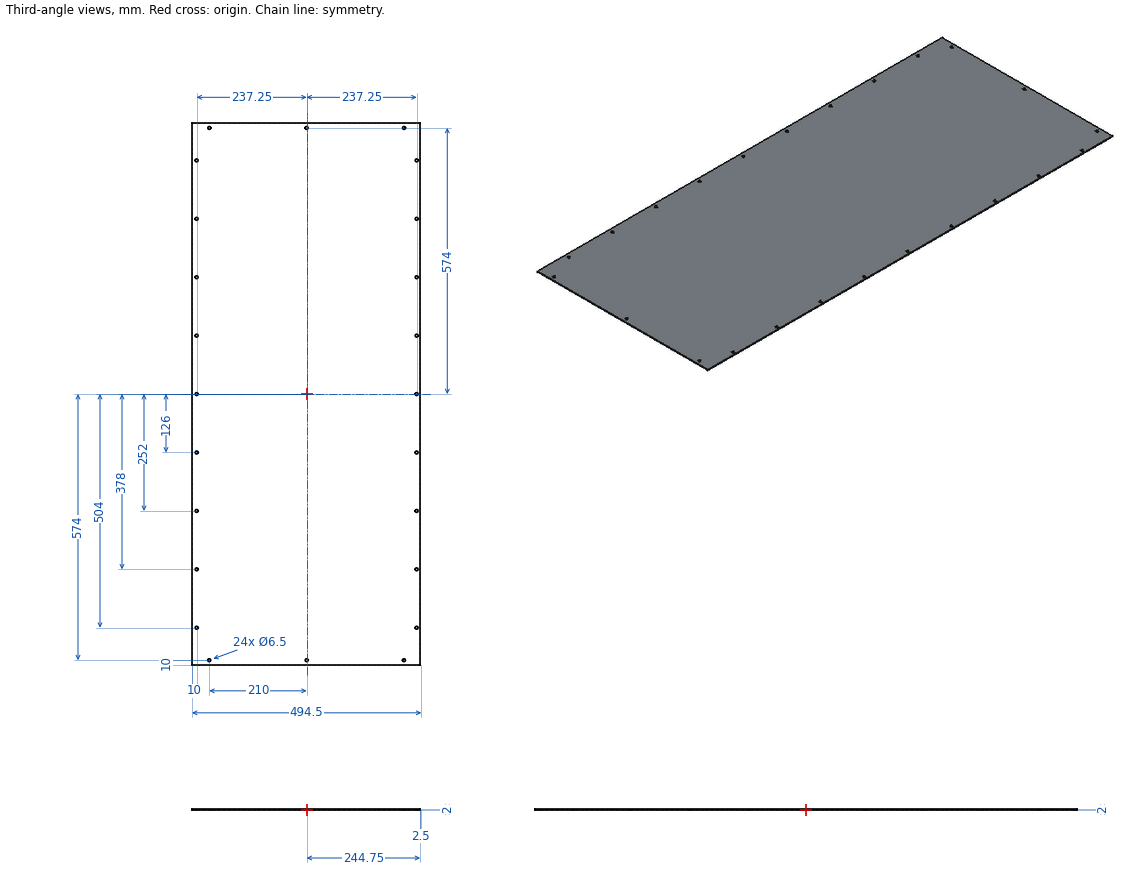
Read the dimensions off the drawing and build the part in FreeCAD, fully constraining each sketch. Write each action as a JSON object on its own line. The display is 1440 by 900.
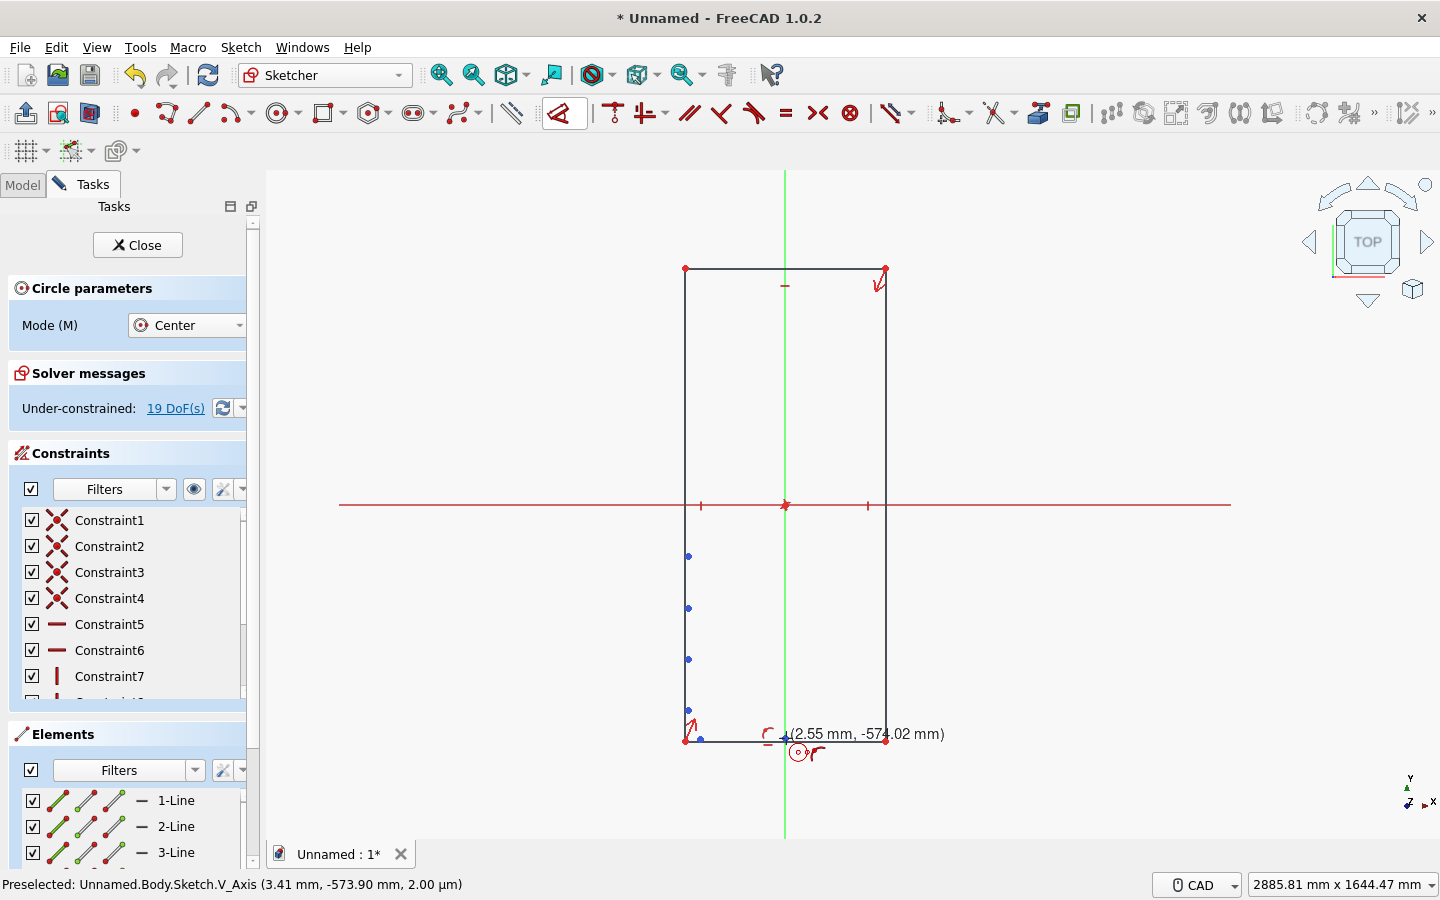
{"action": "scroll", "coordinate": [871, 739], "scroll_direction": "up", "scroll_amount": 15}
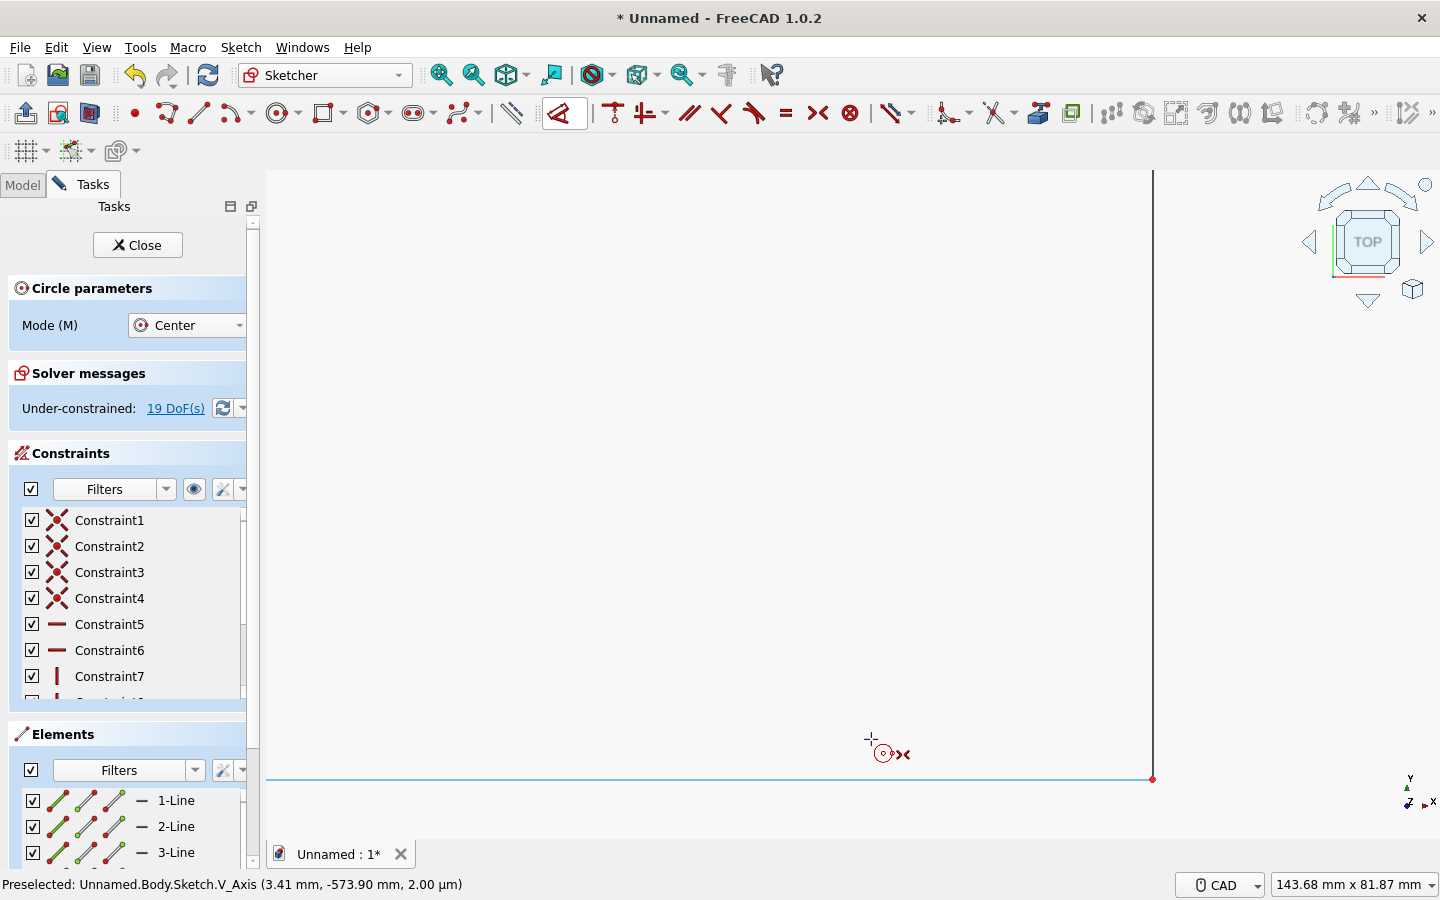
{"action": "scroll", "coordinate": [871, 739], "scroll_direction": "down", "scroll_amount": 15}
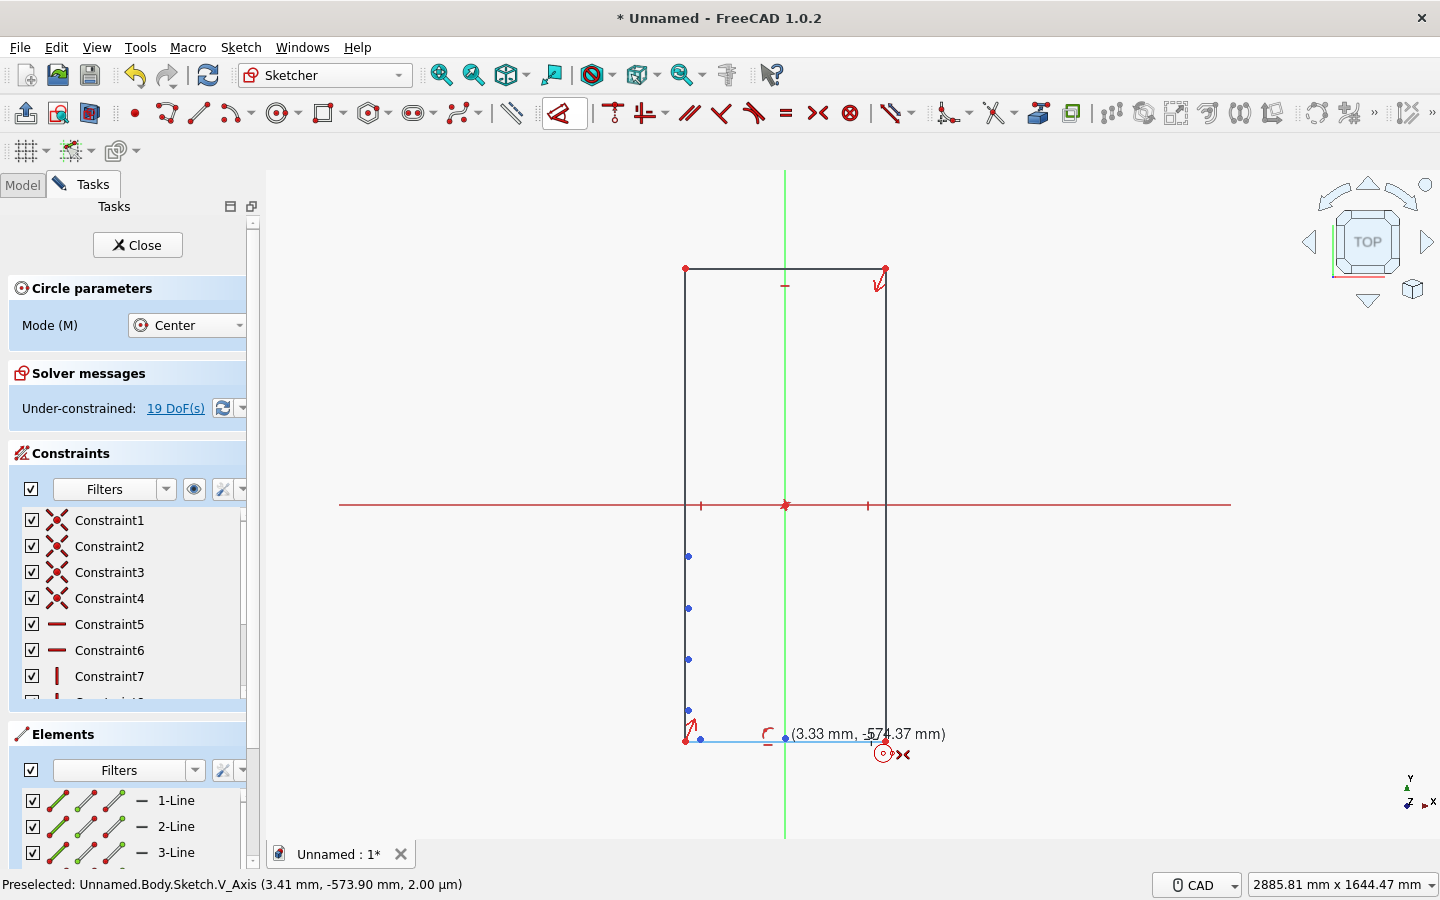
{"action": "scroll", "coordinate": [871, 739], "scroll_direction": "up", "scroll_amount": 7}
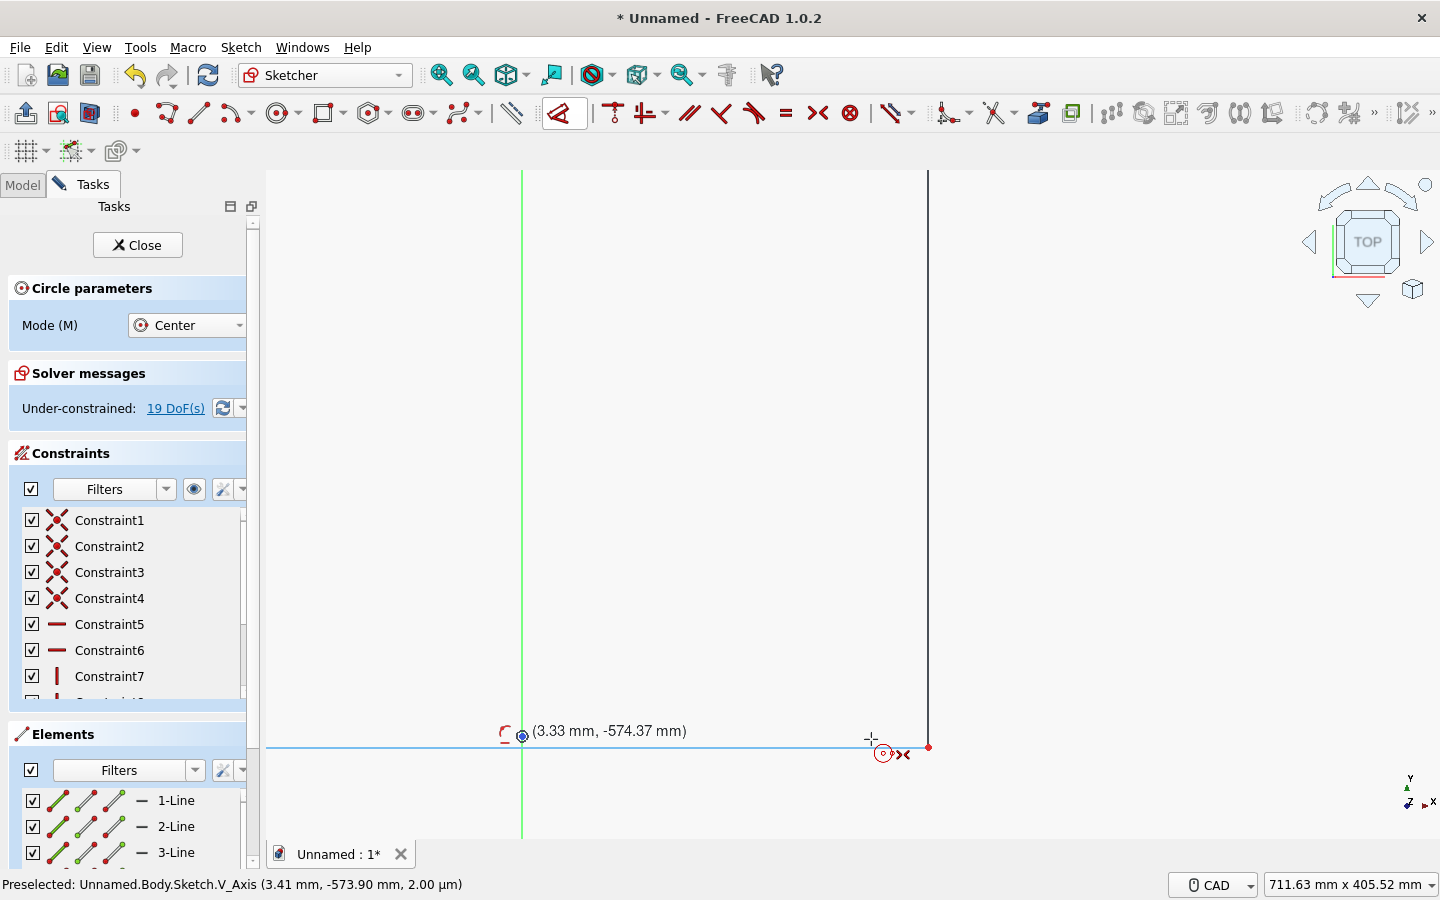
{"action": "left_click", "coordinate": [869, 736]}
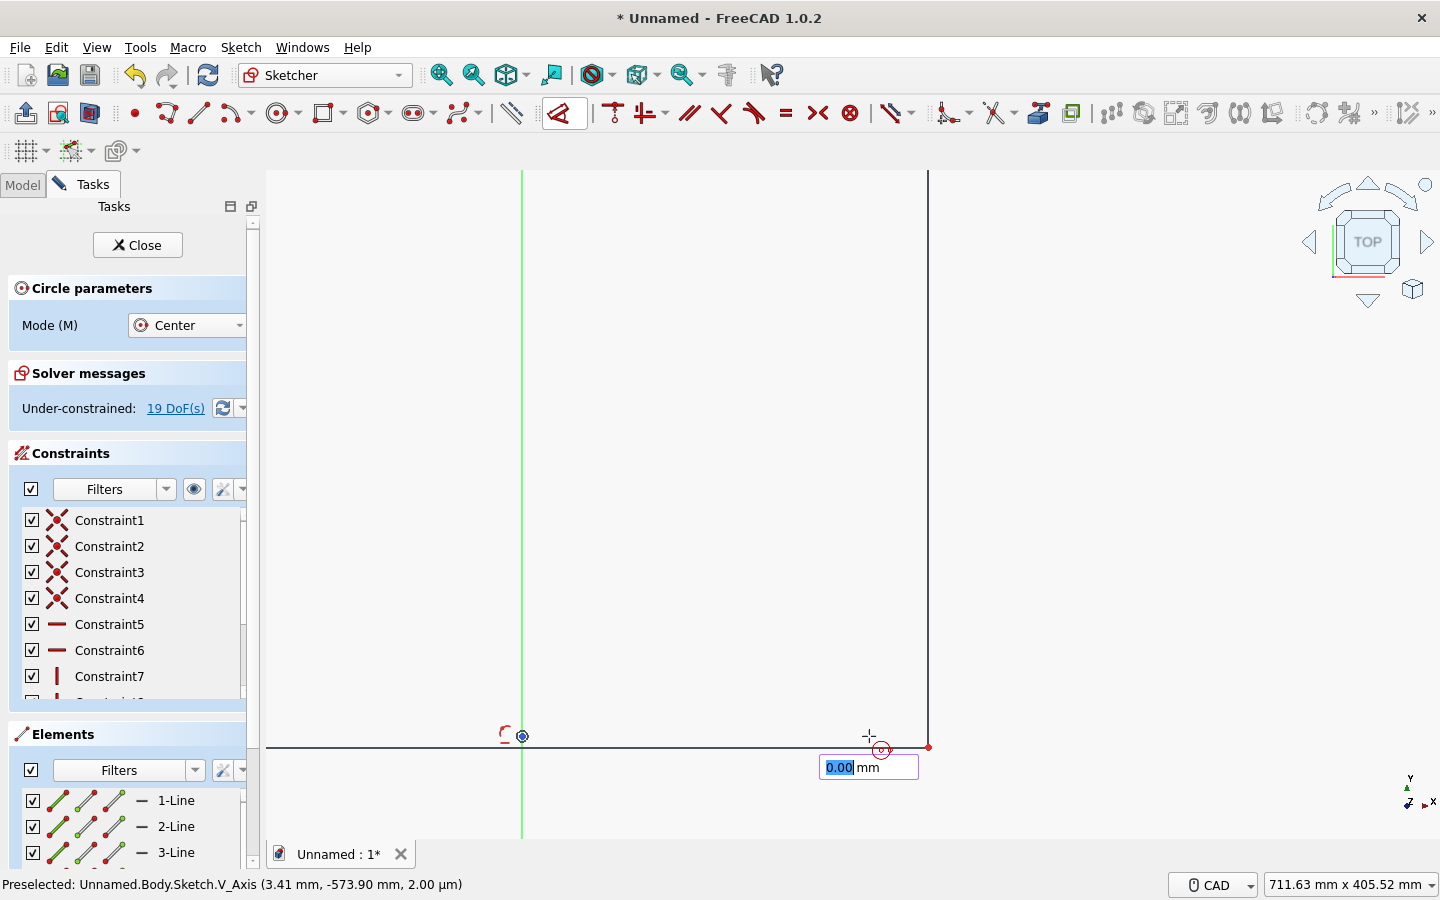
{"action": "scroll", "coordinate": [872, 732], "scroll_direction": "up", "scroll_amount": 6}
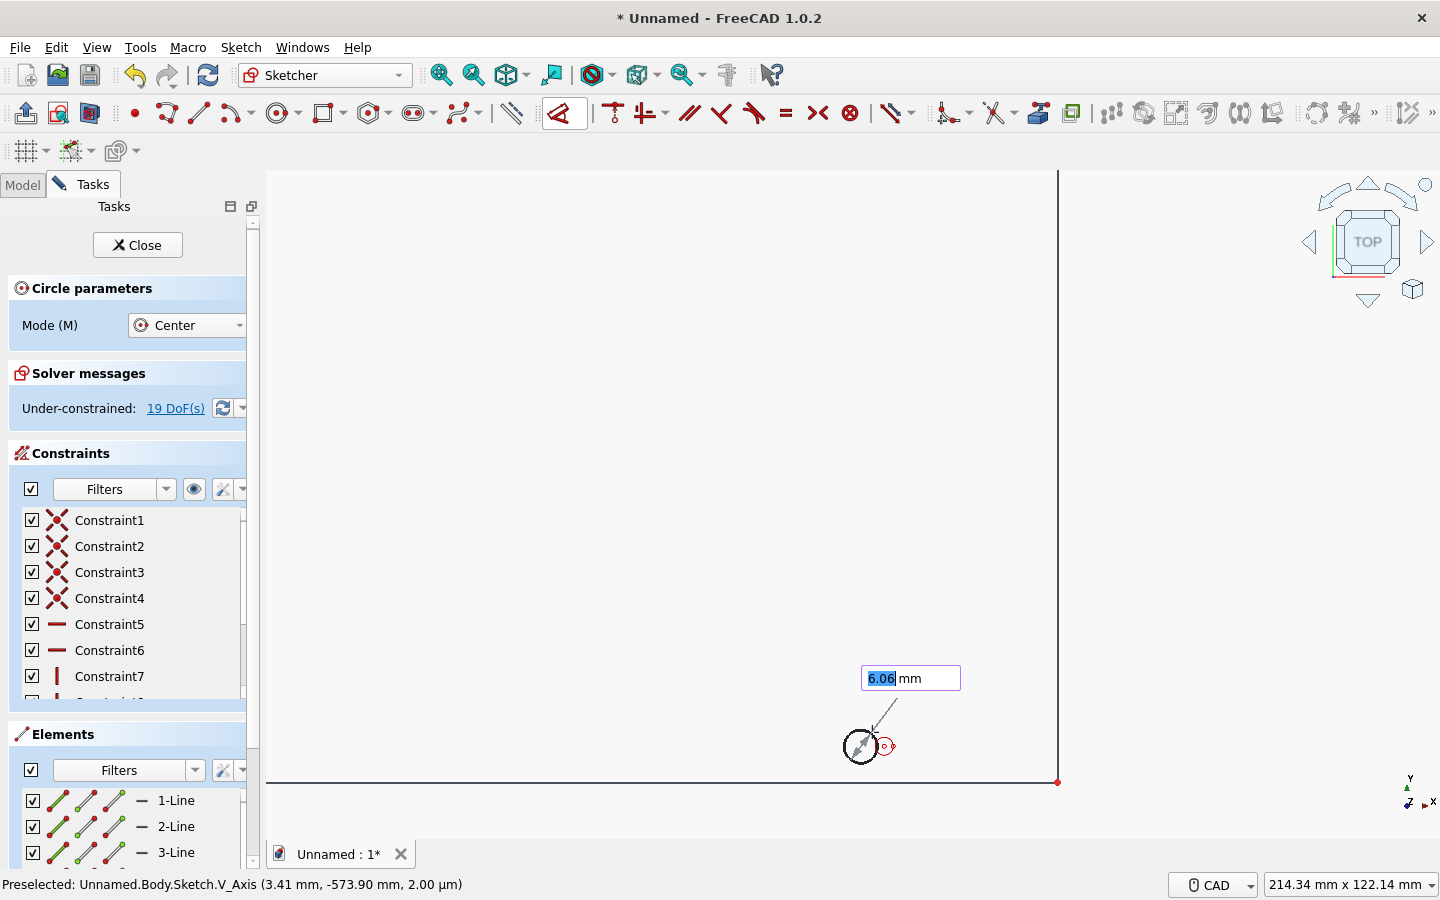
{"action": "left_click", "coordinate": [872, 730]}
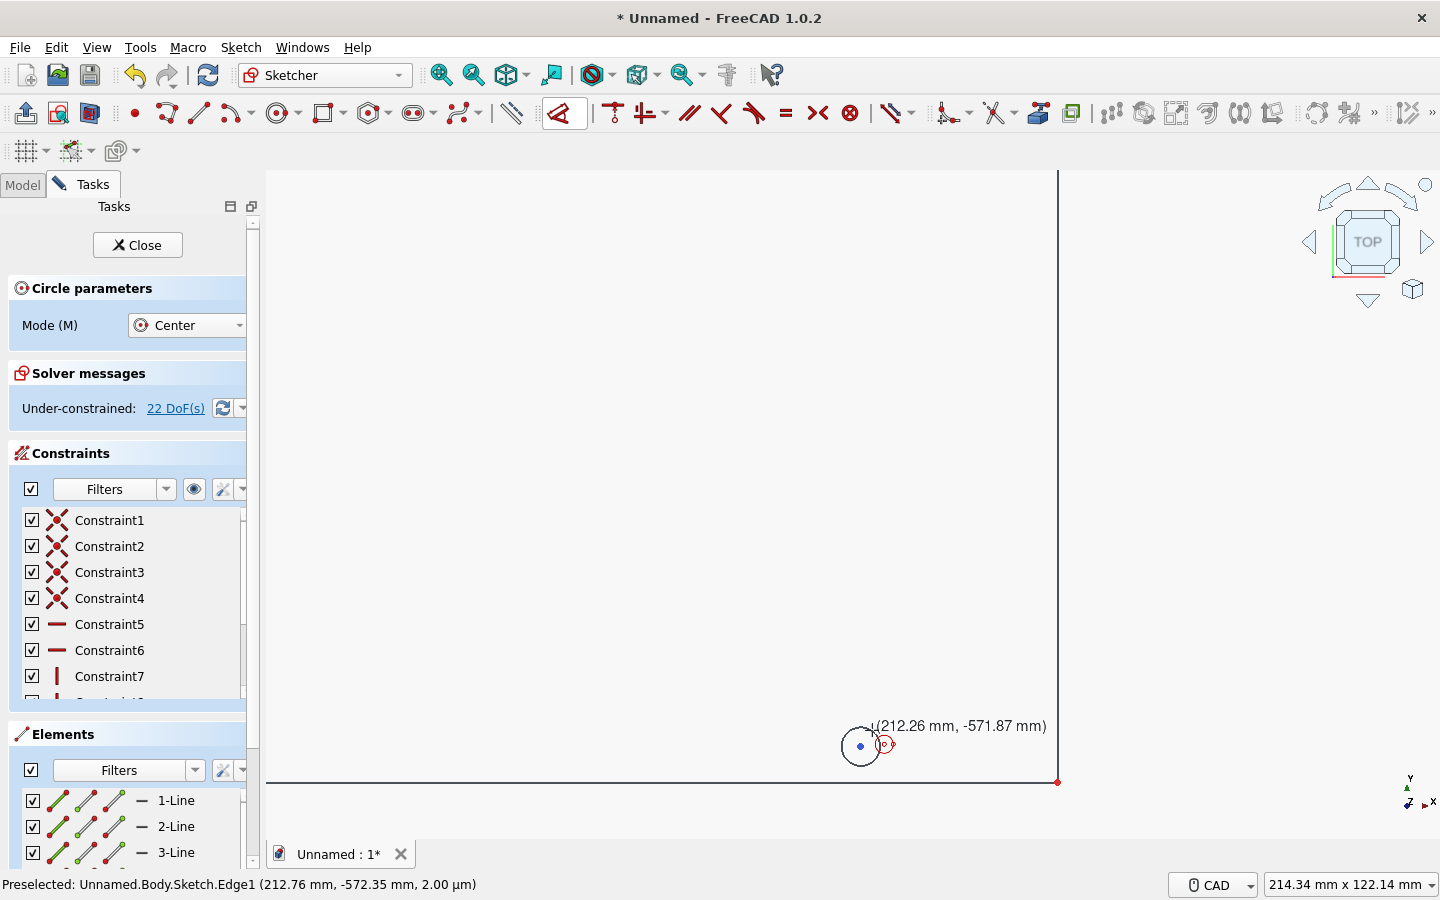
{"action": "scroll", "coordinate": [1009, 359], "scroll_direction": "up", "scroll_amount": 2}